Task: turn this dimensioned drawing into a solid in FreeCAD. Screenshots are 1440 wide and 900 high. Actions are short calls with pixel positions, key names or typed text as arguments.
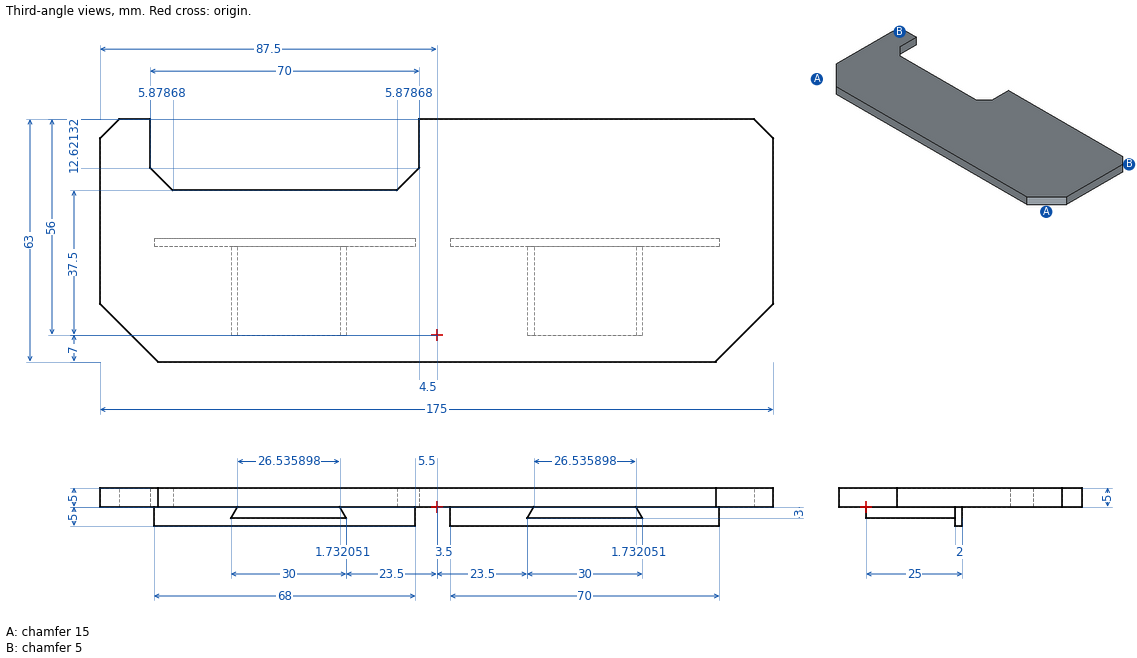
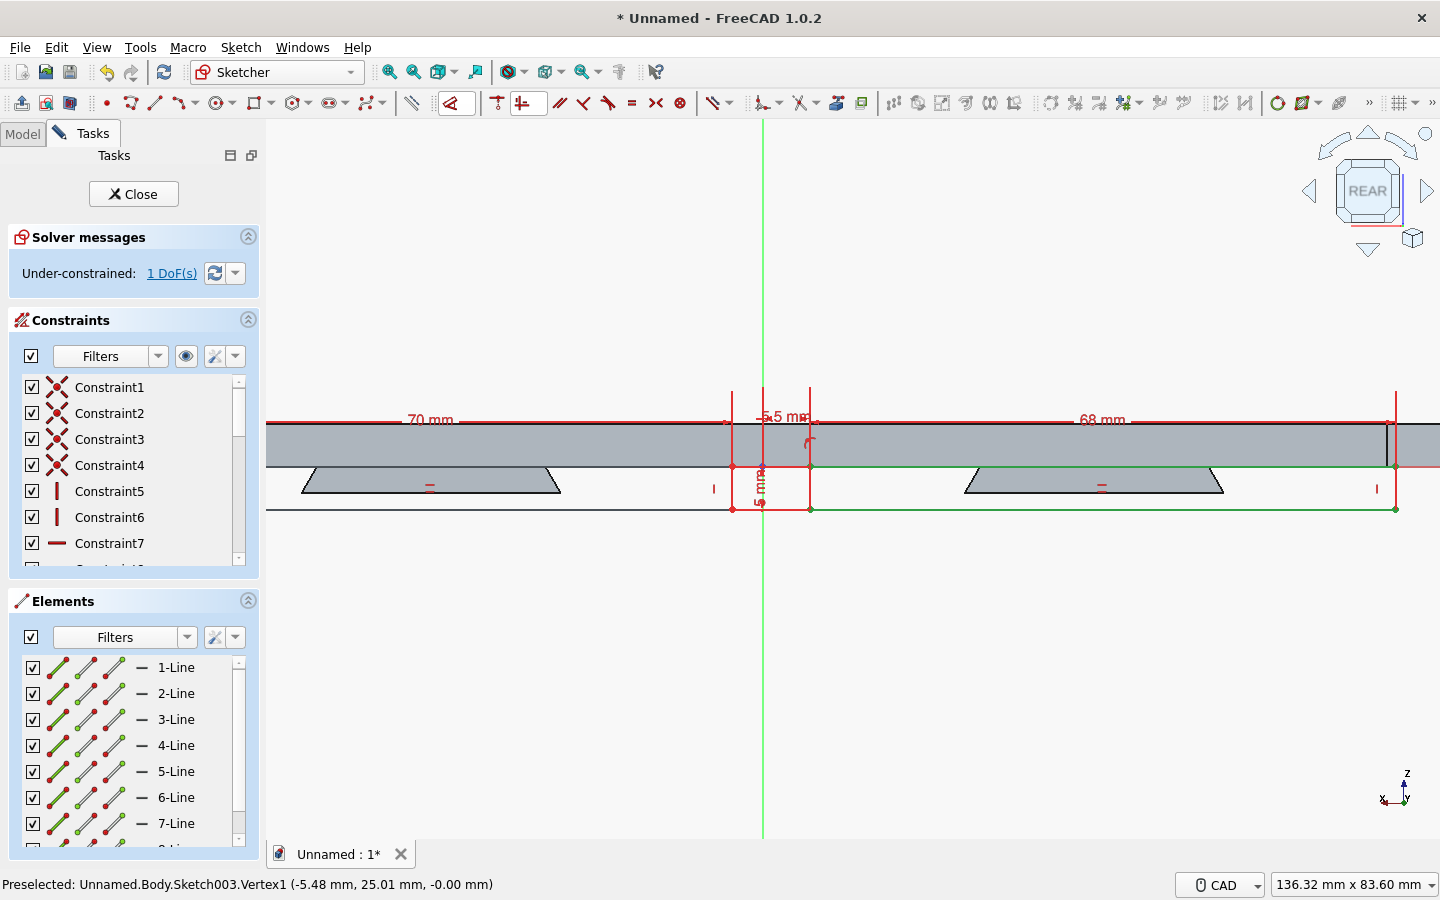
scroll(732, 510, up, 2)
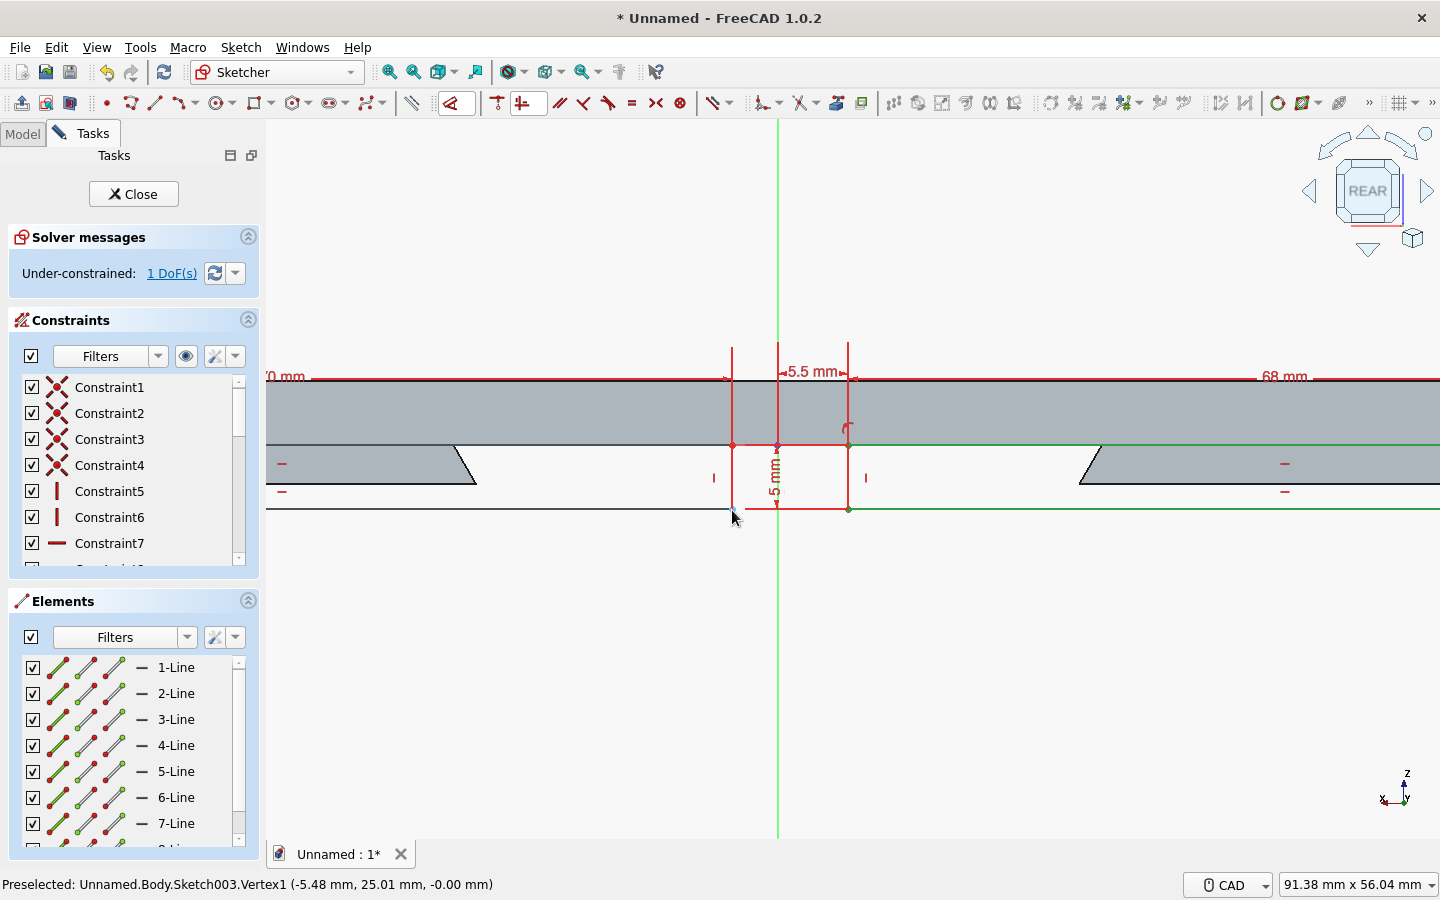
click(732, 509)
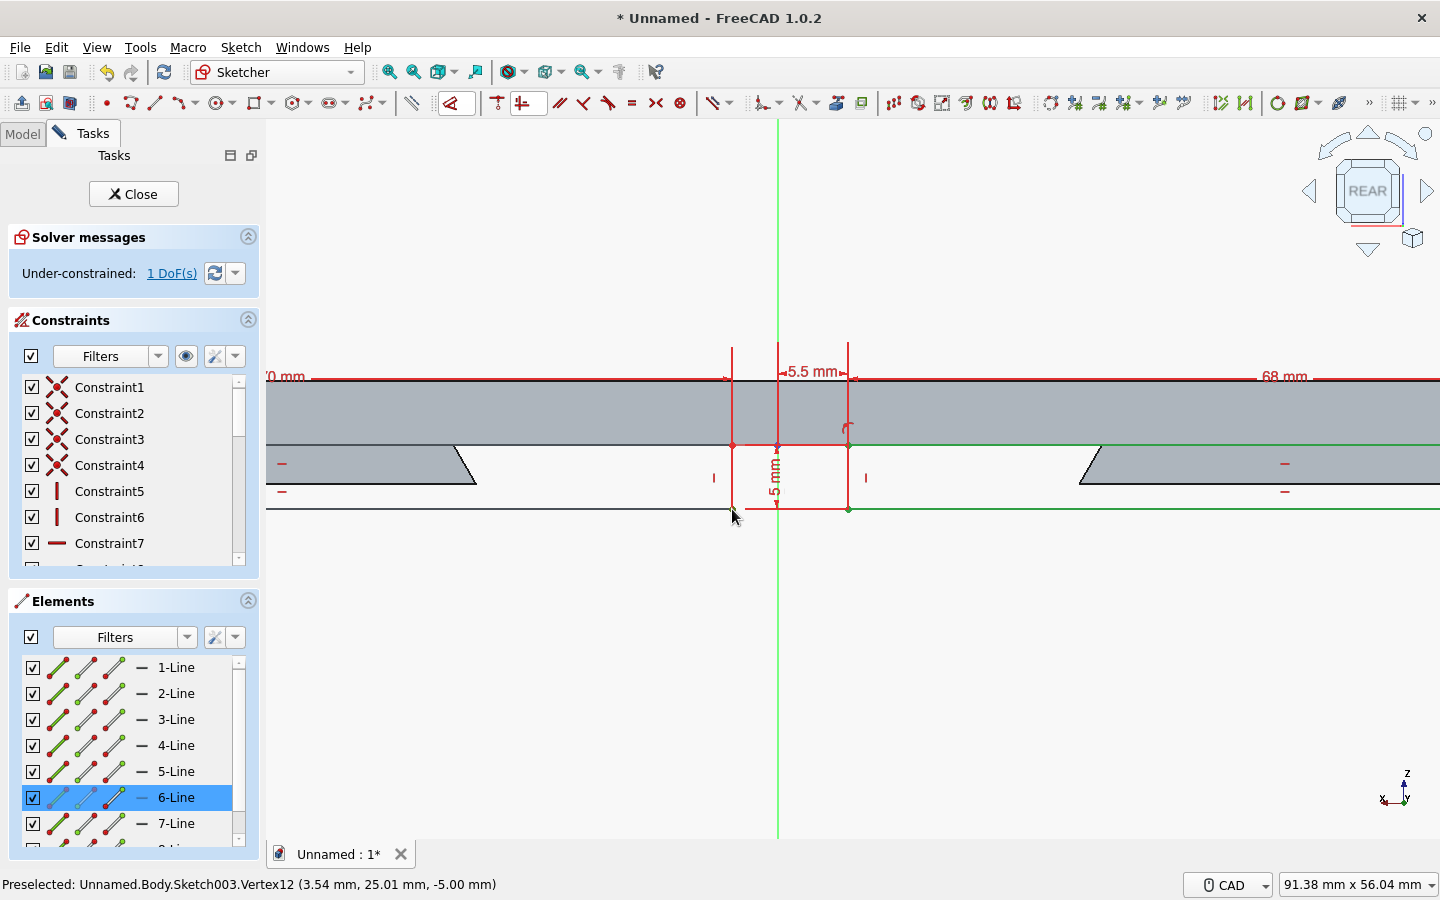
key(l)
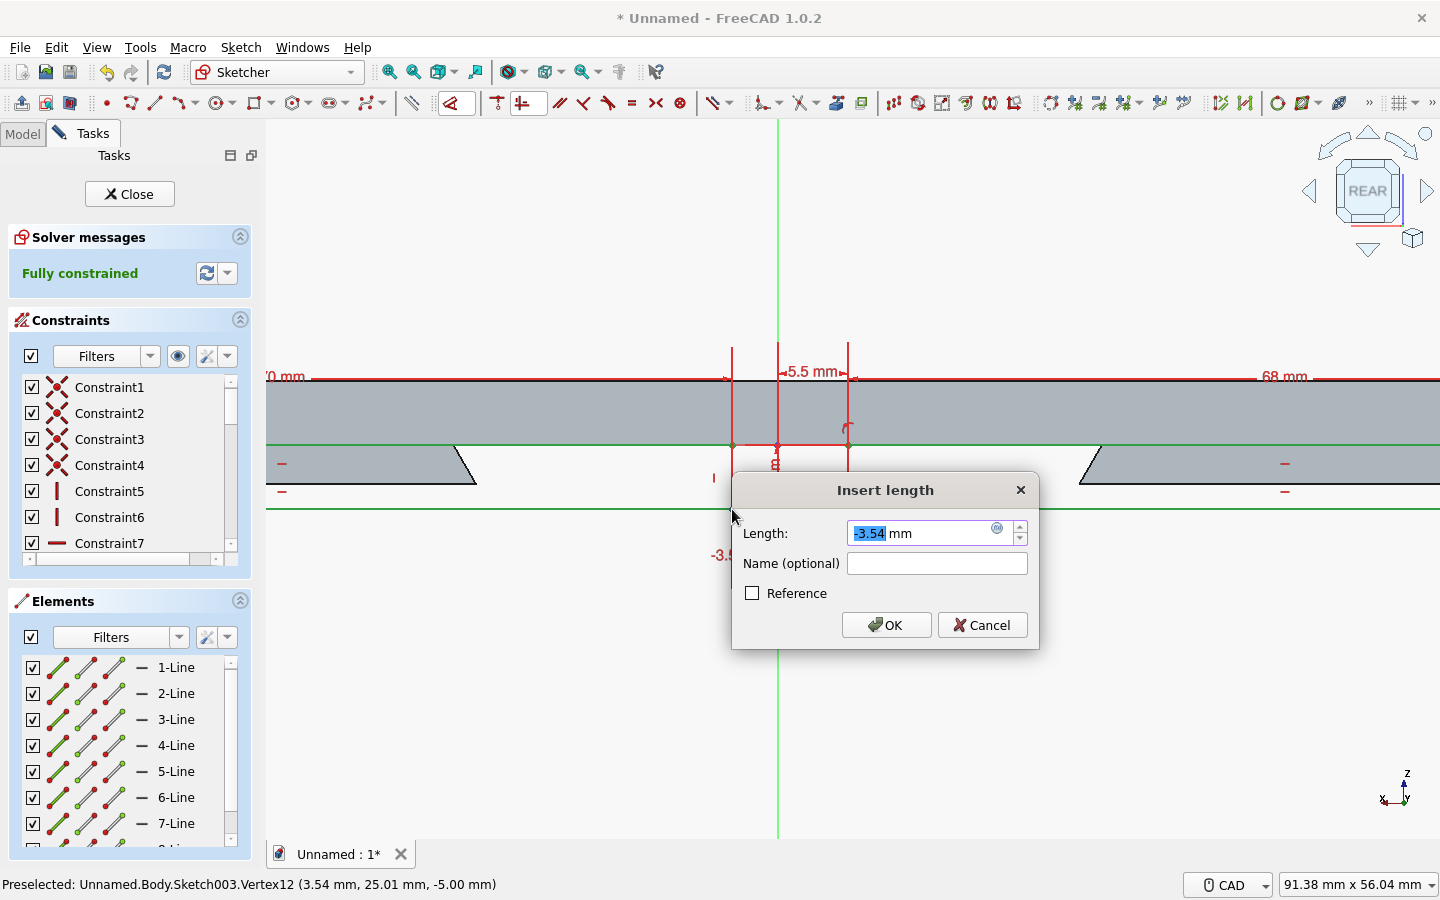
text(-3.5)
key(Return)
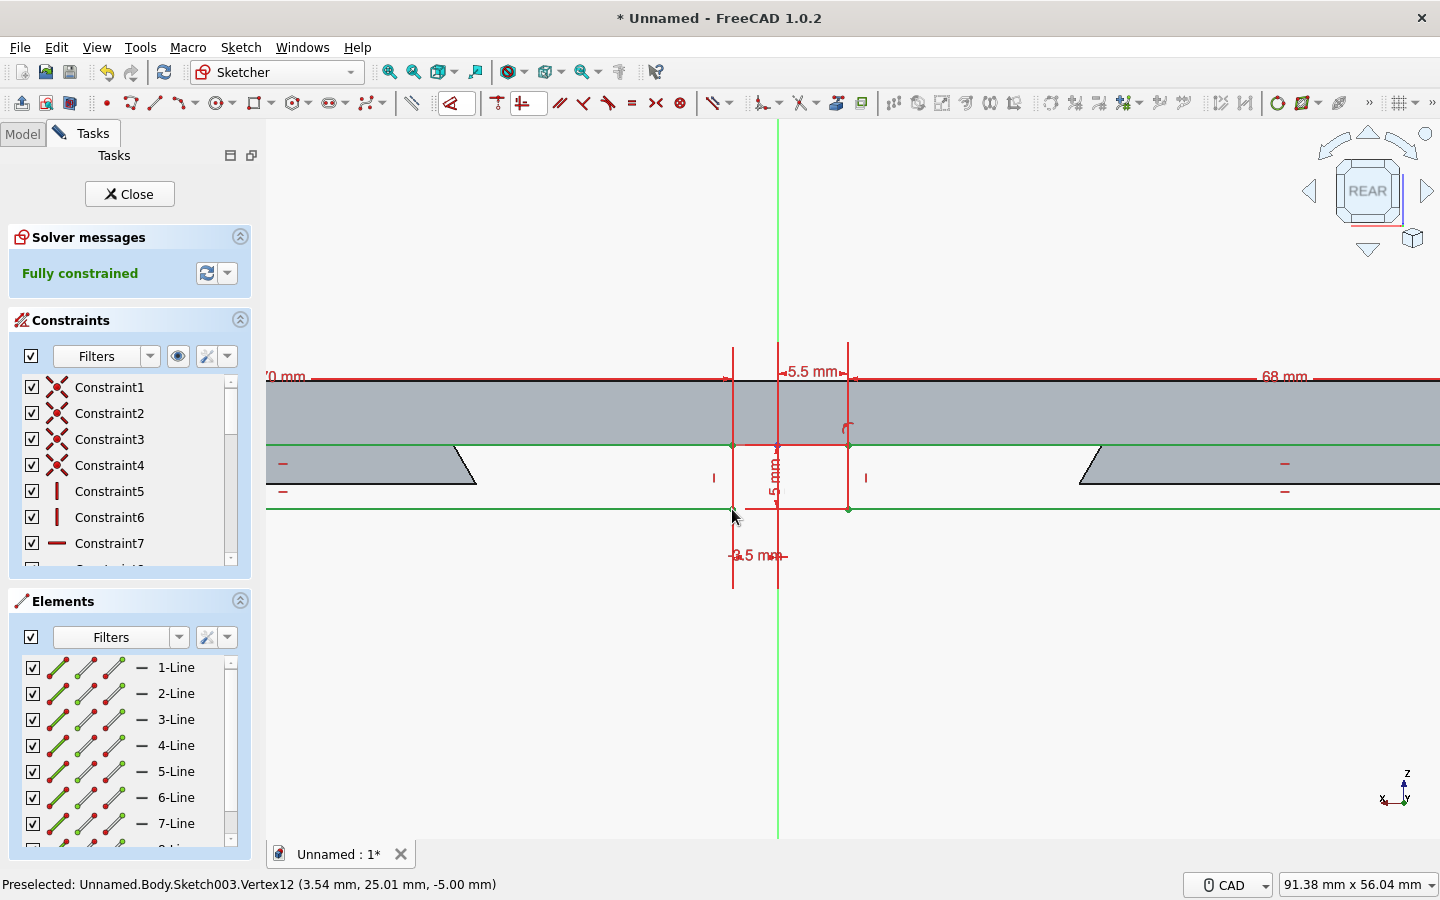
click(130, 194)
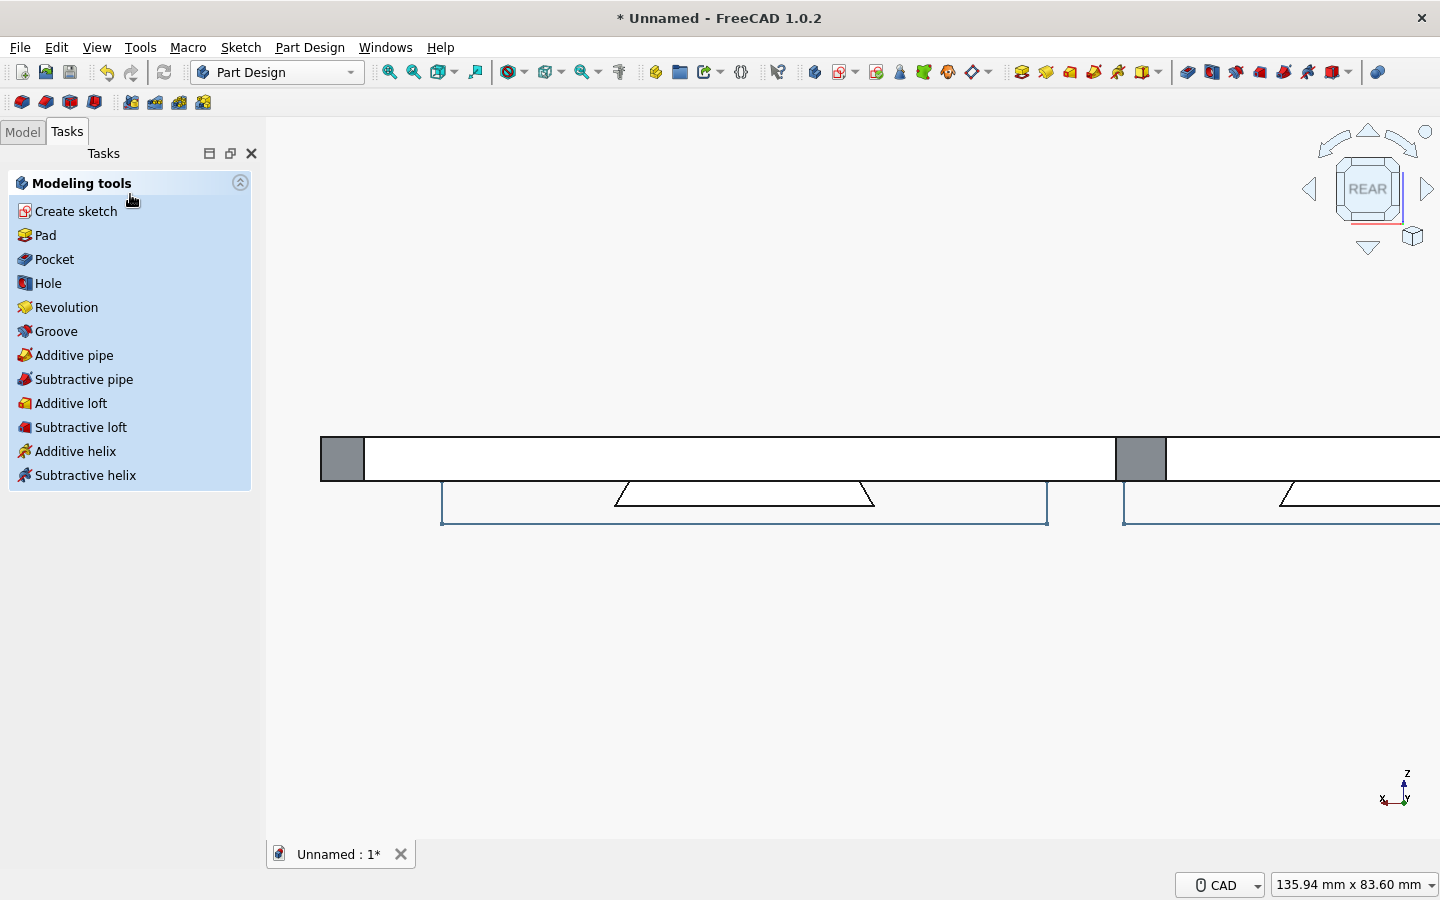
click(1022, 72)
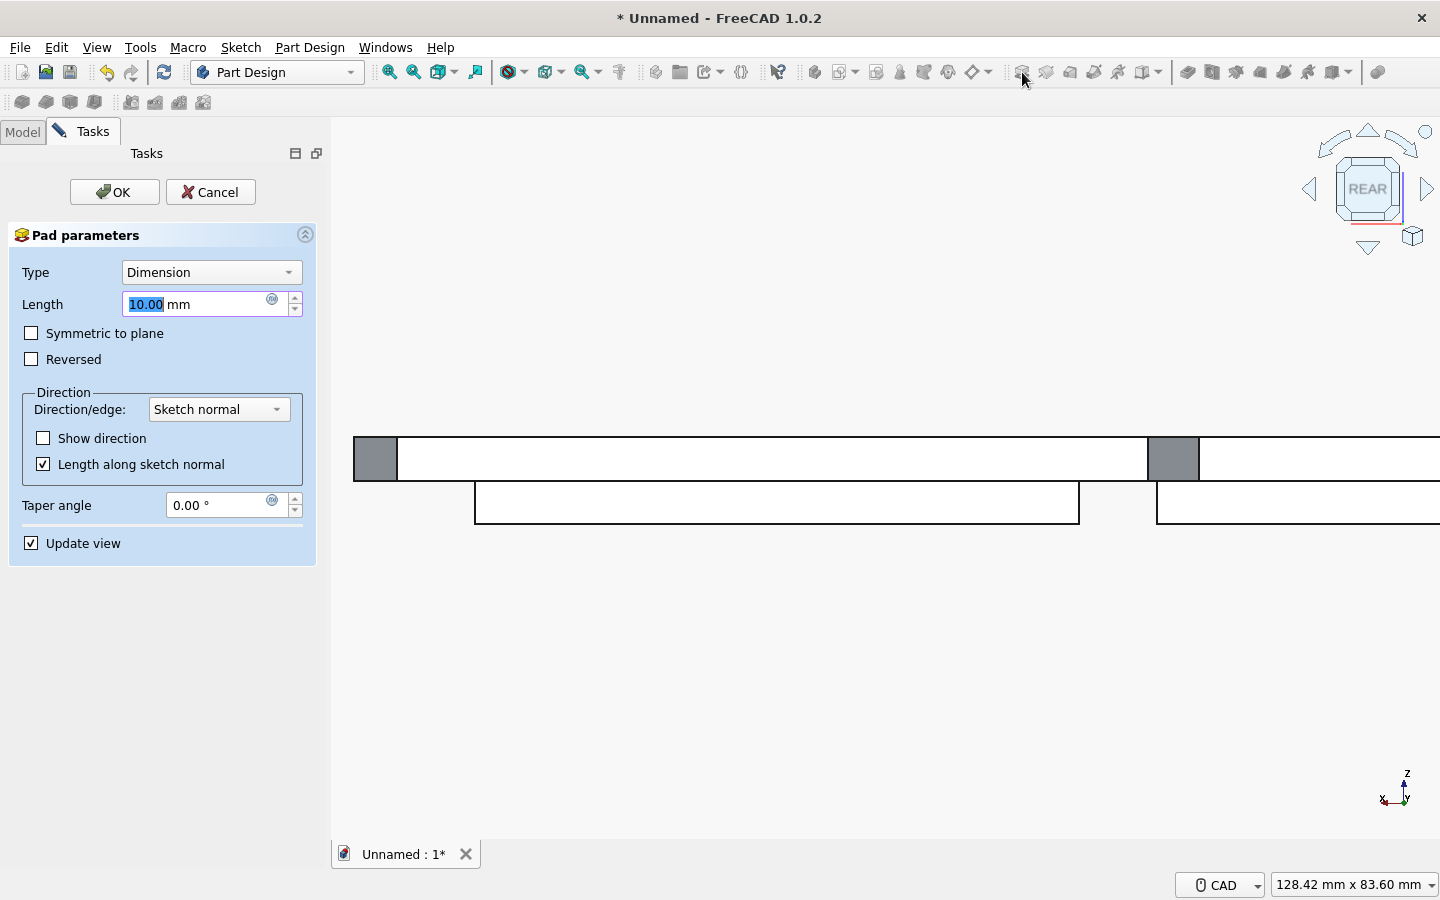
text(2)
key(Tab)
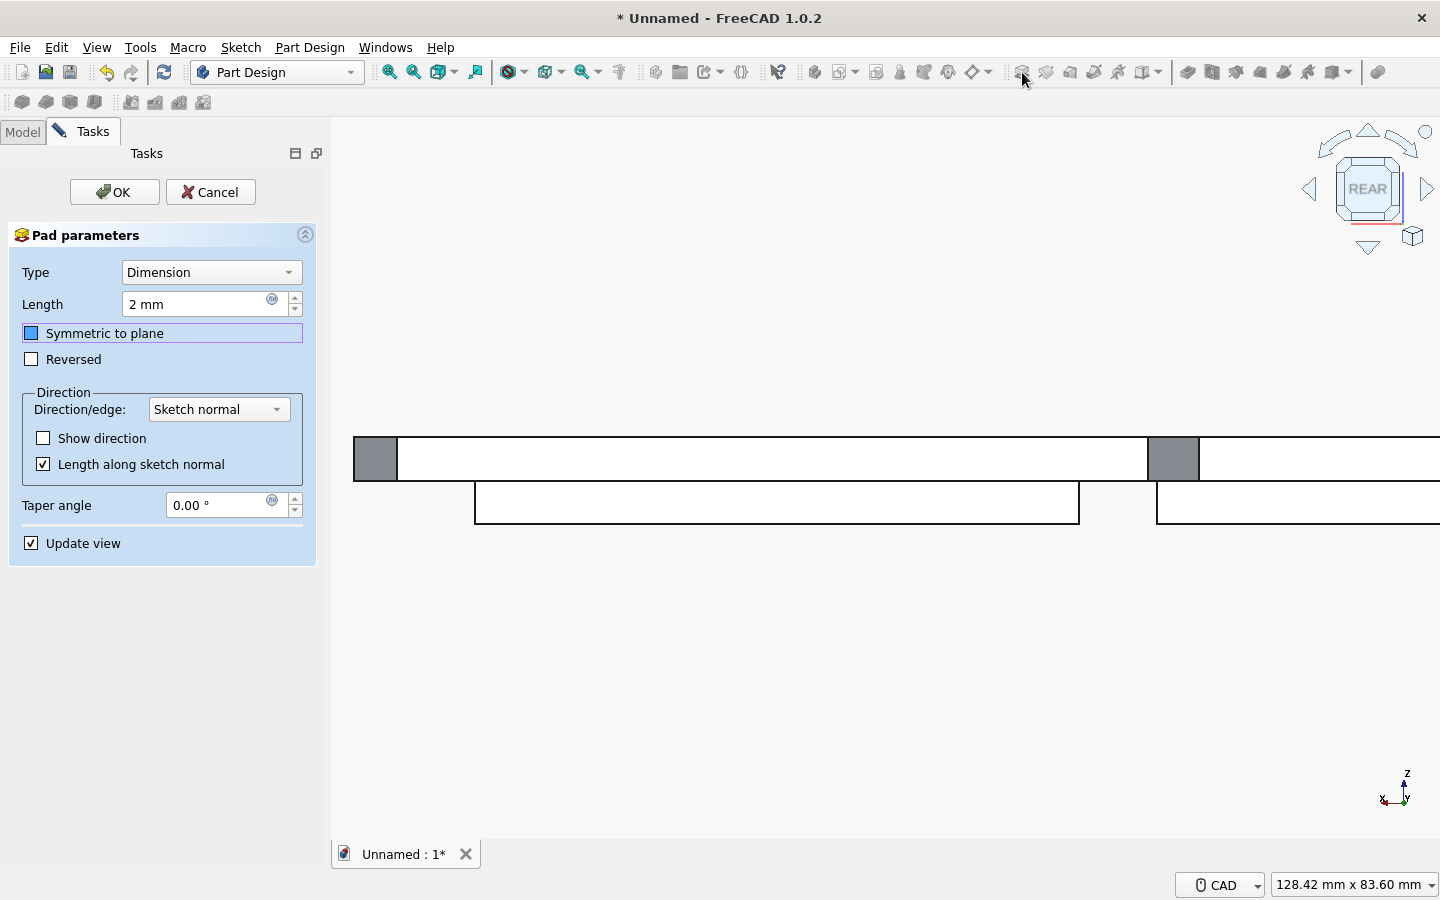
click(30, 359)